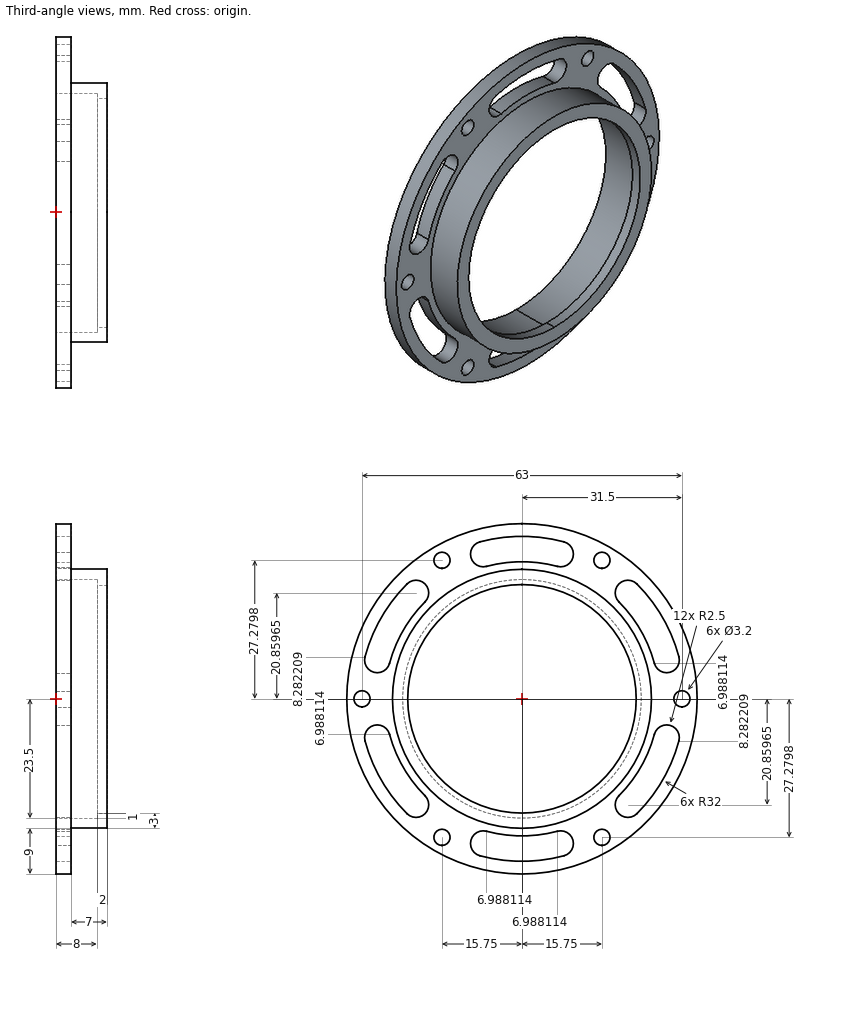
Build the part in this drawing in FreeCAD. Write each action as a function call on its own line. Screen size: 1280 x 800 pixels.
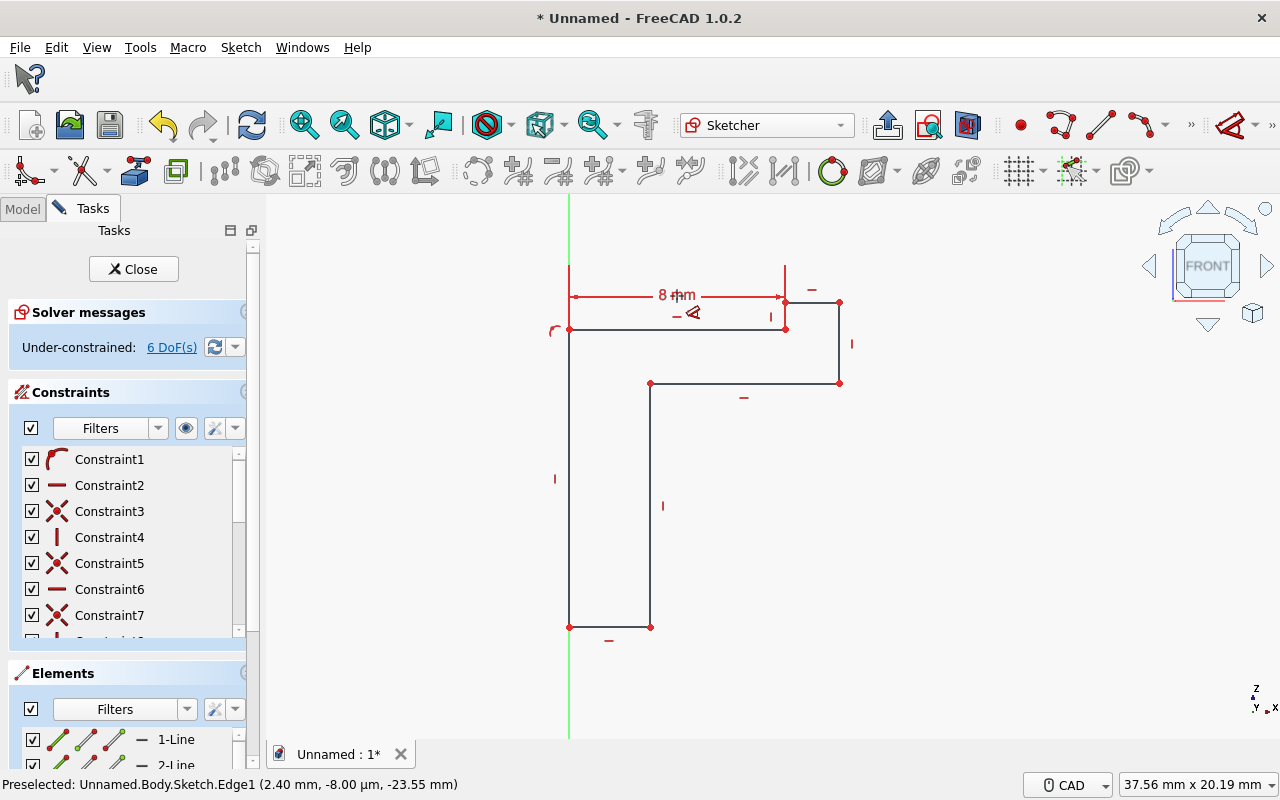
scroll(785, 319, up, 2)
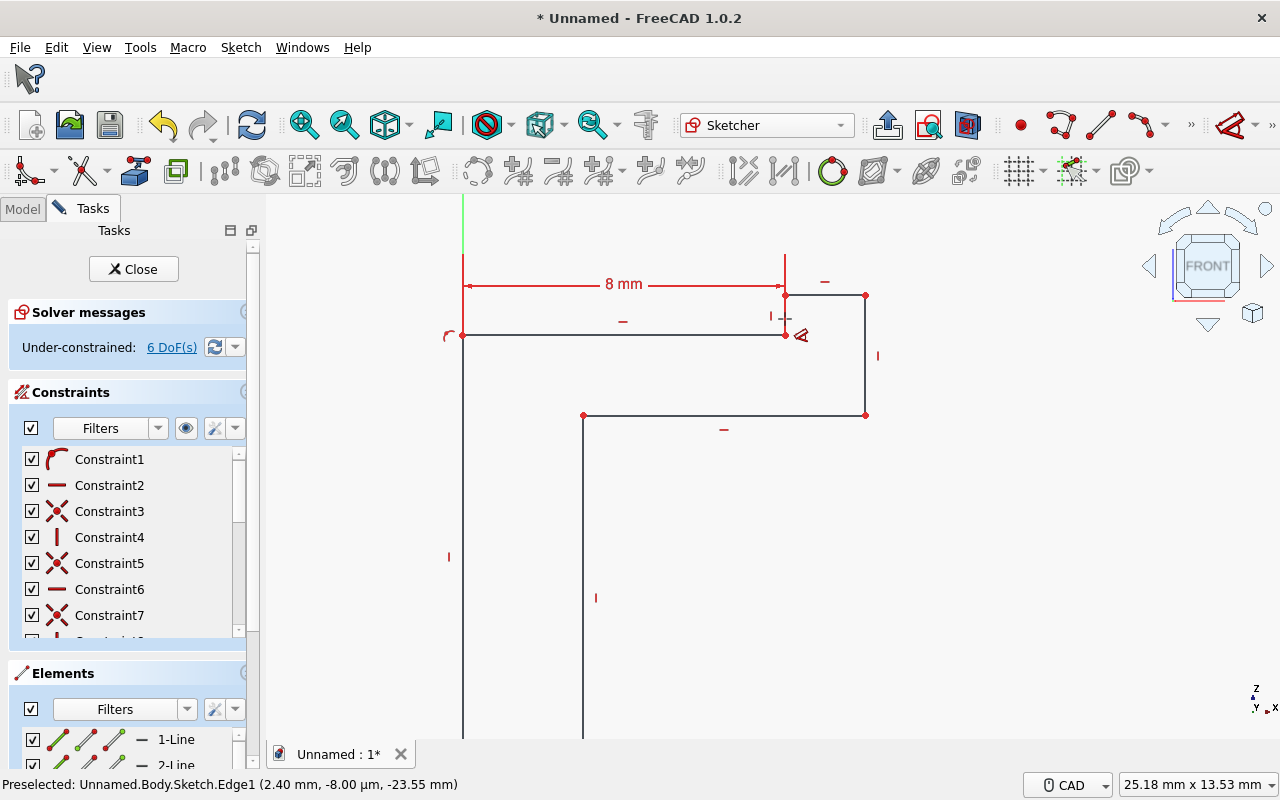
click(785, 319)
click(819, 315)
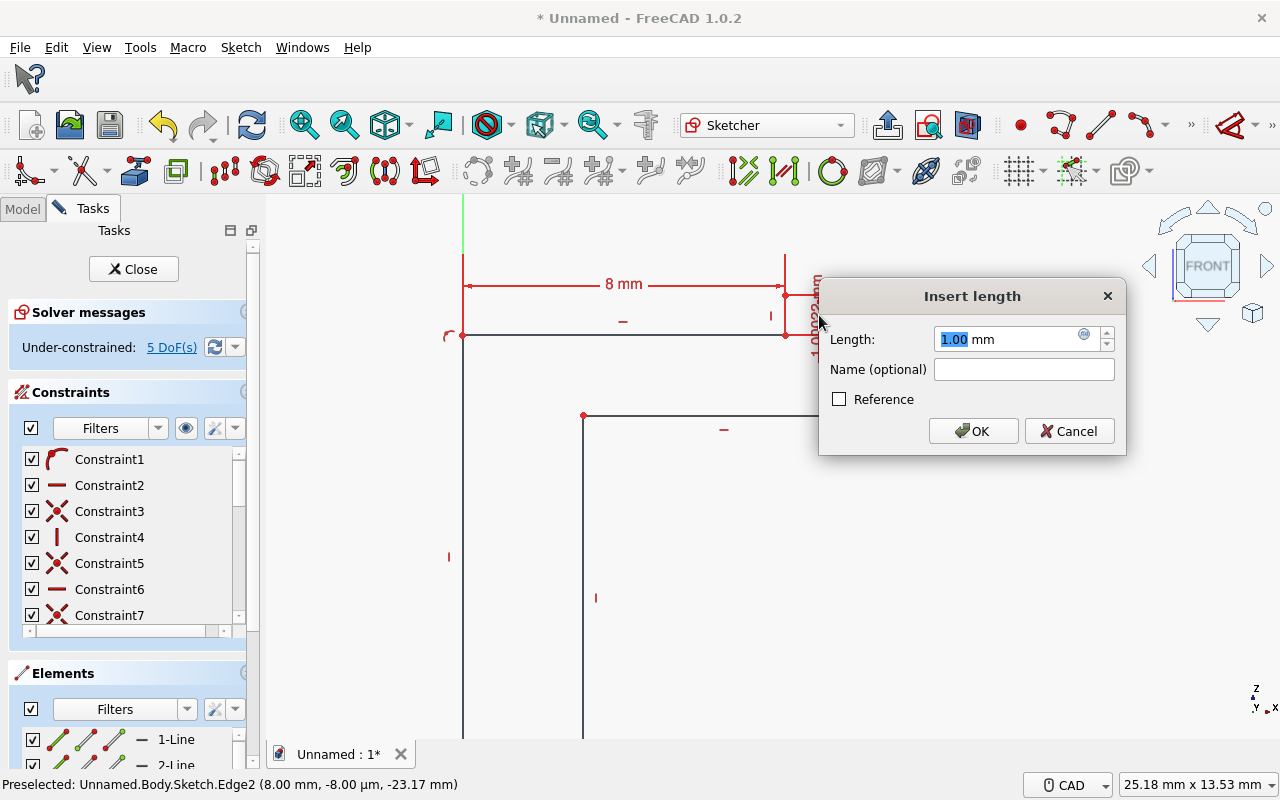
text(1)
key(Return)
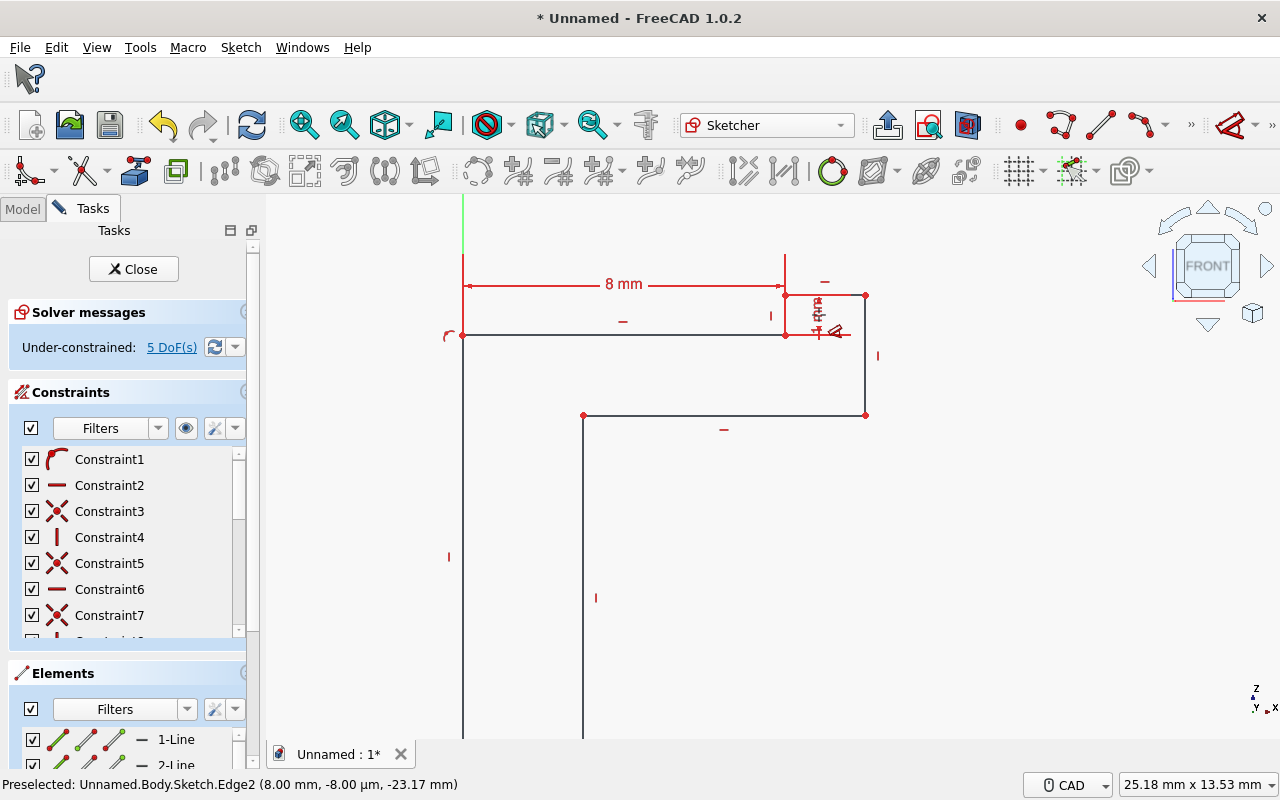
click(809, 295)
click(825, 261)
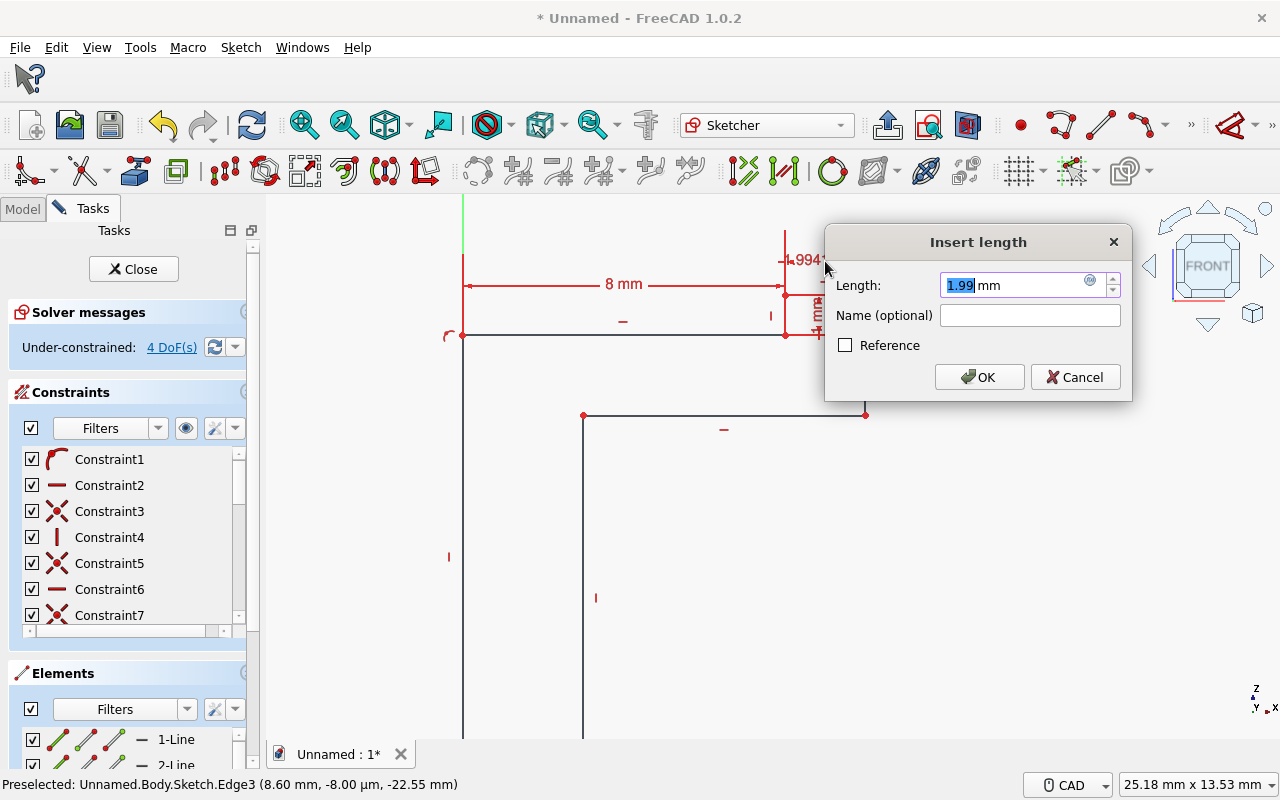
text(2)
key(Return)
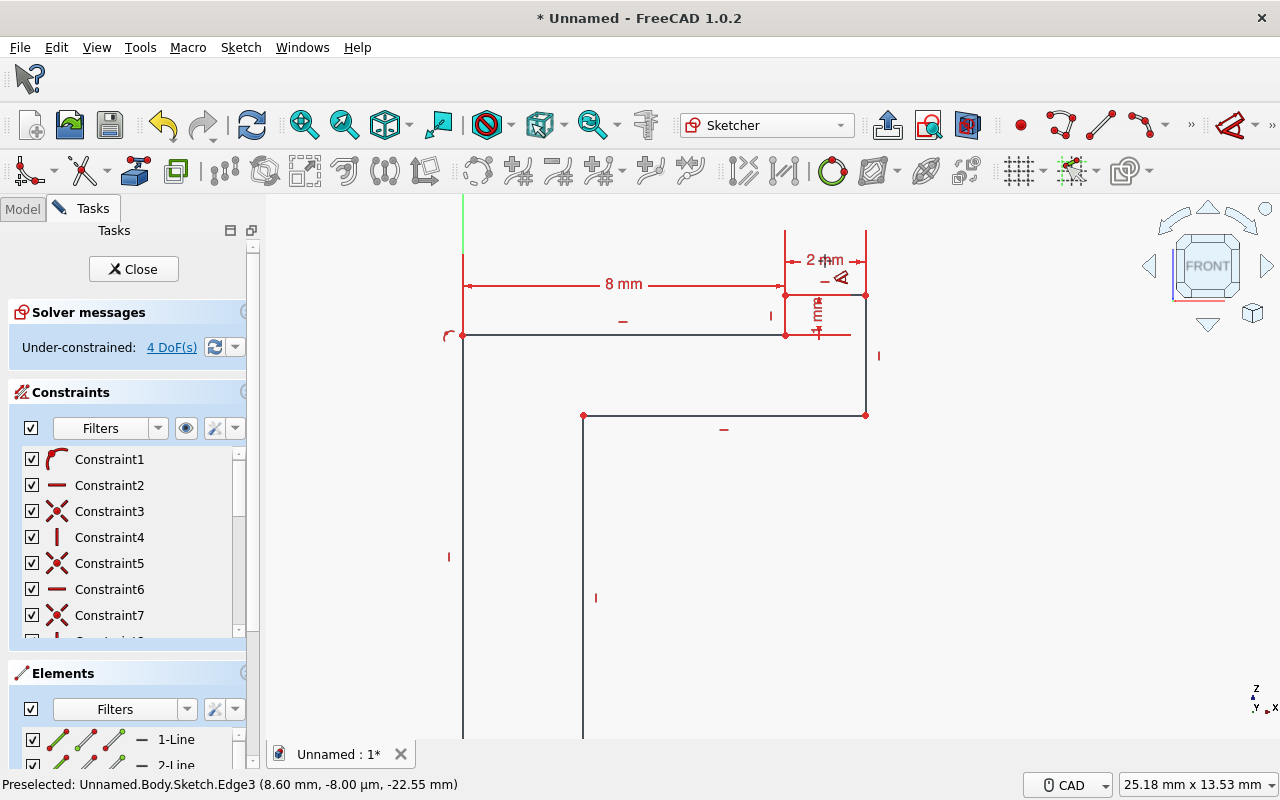
click(866, 331)
click(900, 355)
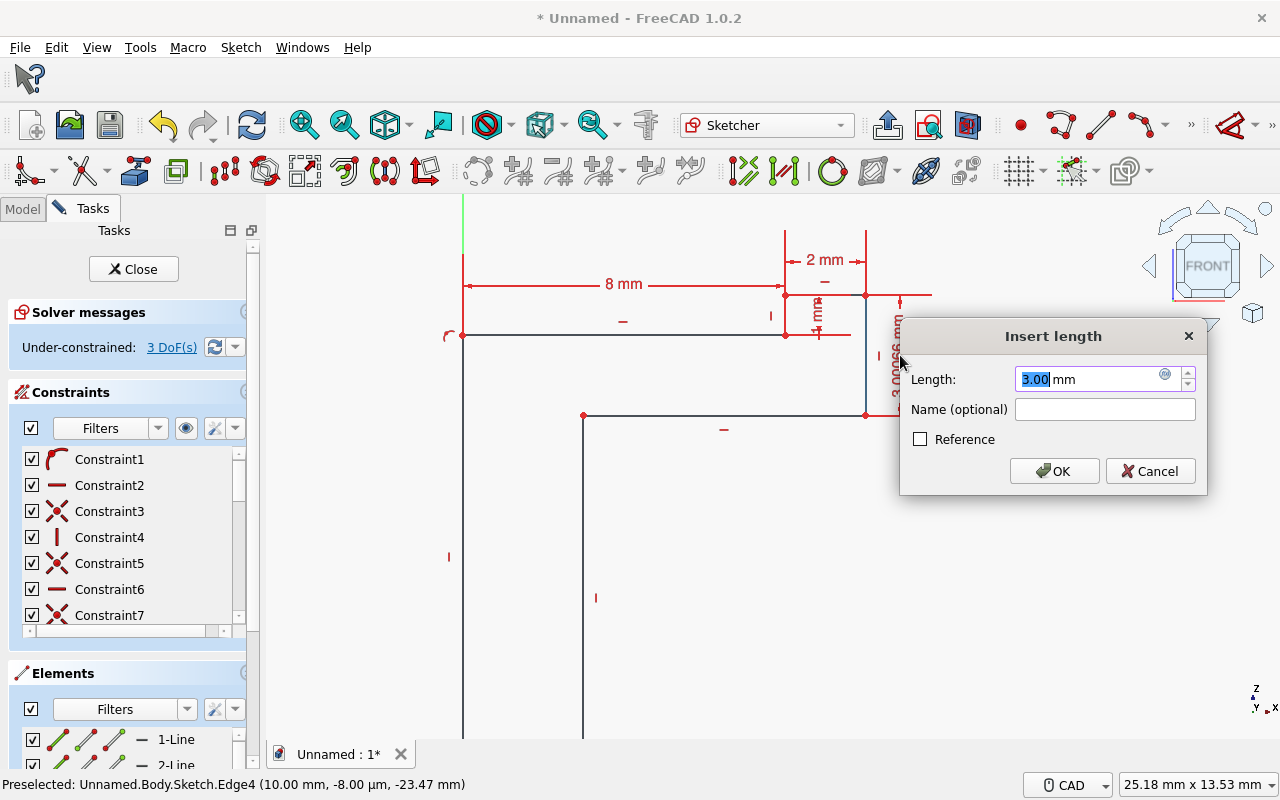
text(3)
key(Return)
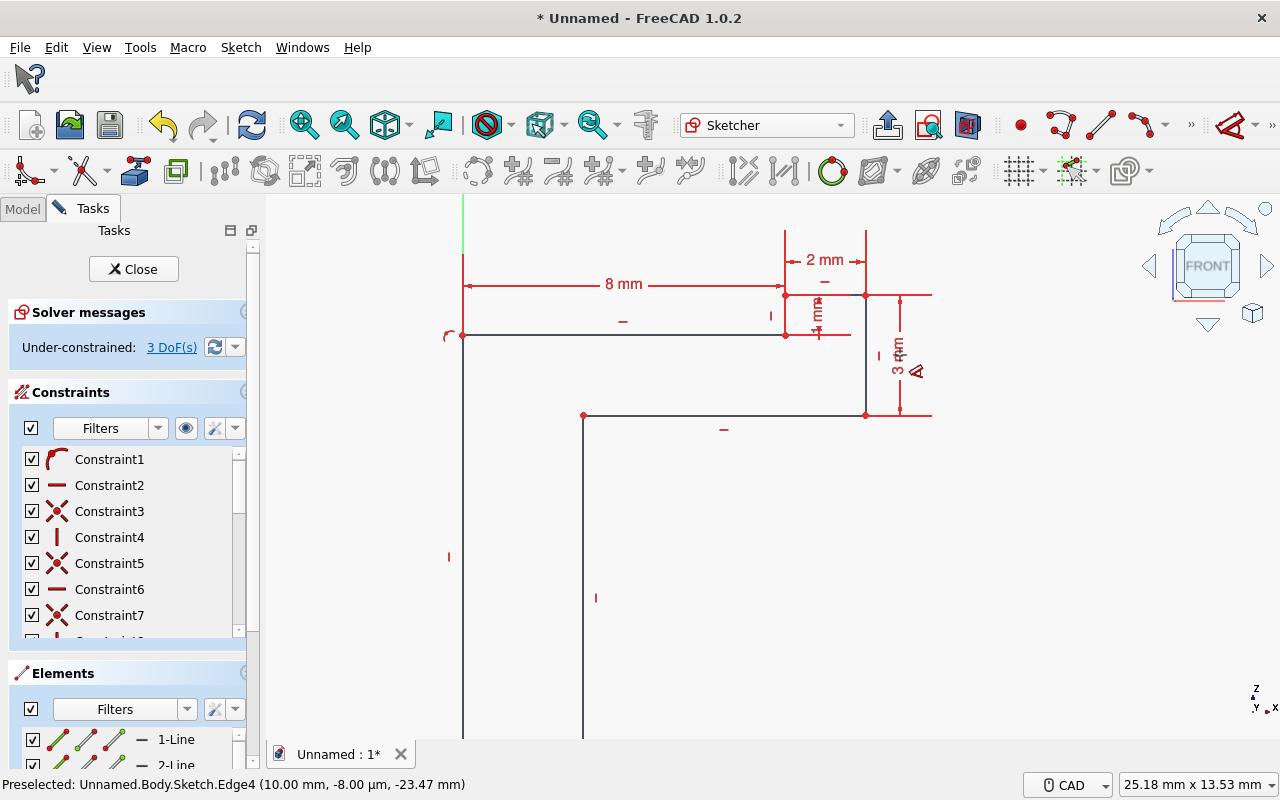
click(781, 416)
click(724, 382)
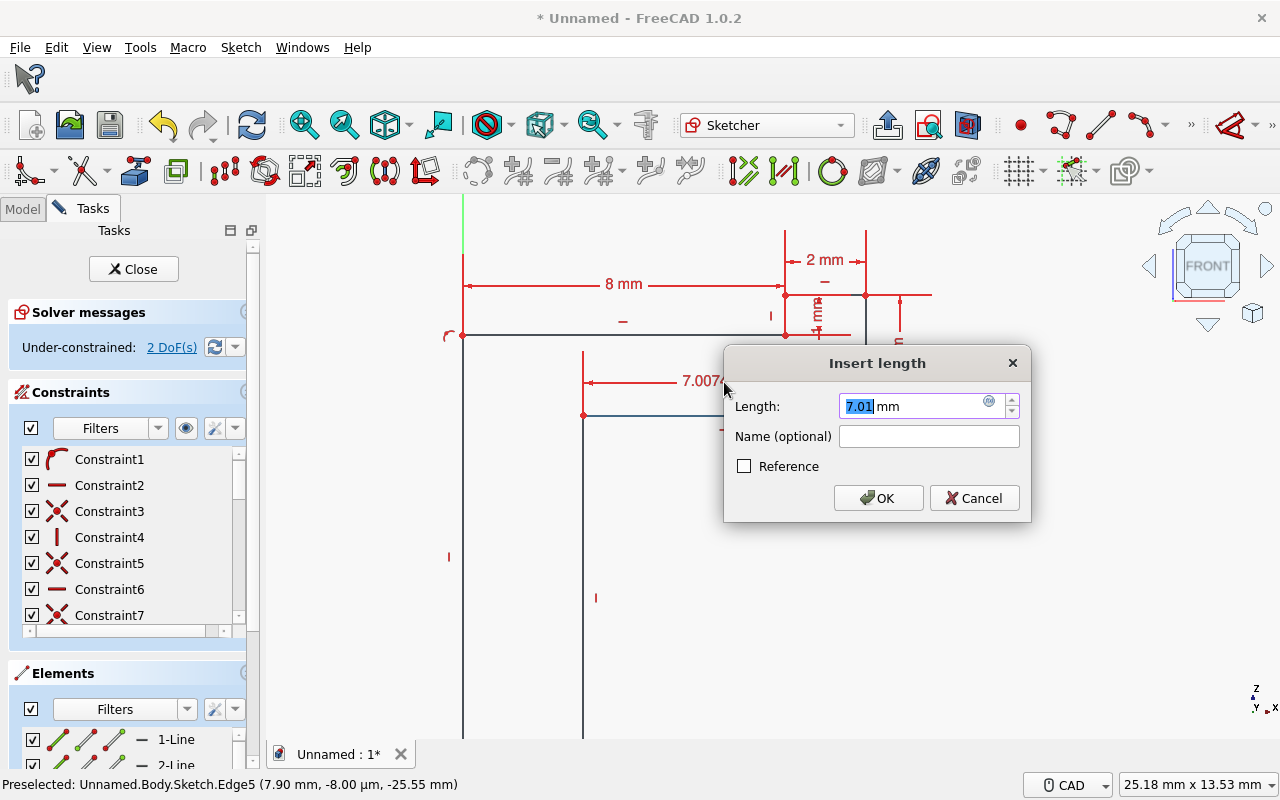
text(7)
key(Return)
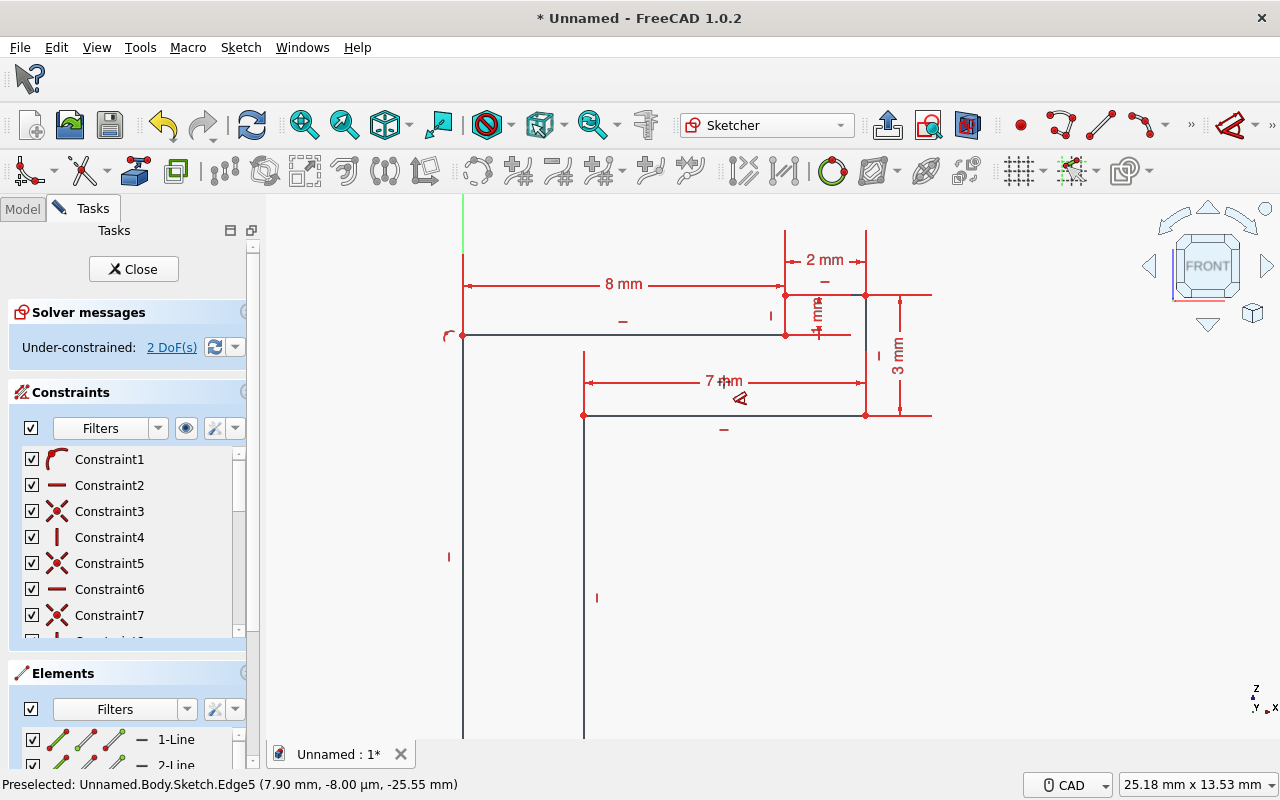
click(584, 525)
click(550, 563)